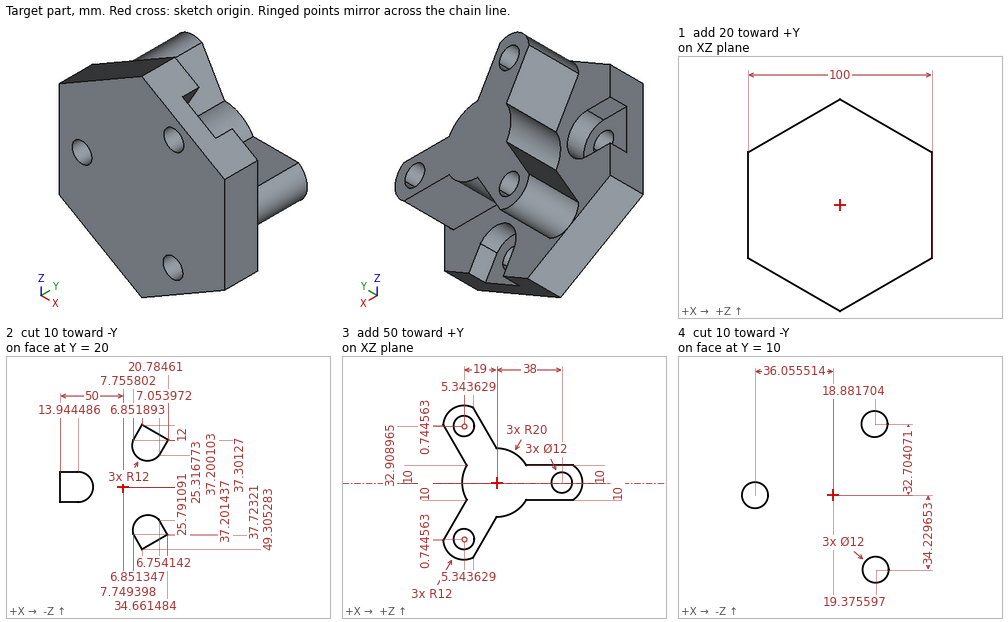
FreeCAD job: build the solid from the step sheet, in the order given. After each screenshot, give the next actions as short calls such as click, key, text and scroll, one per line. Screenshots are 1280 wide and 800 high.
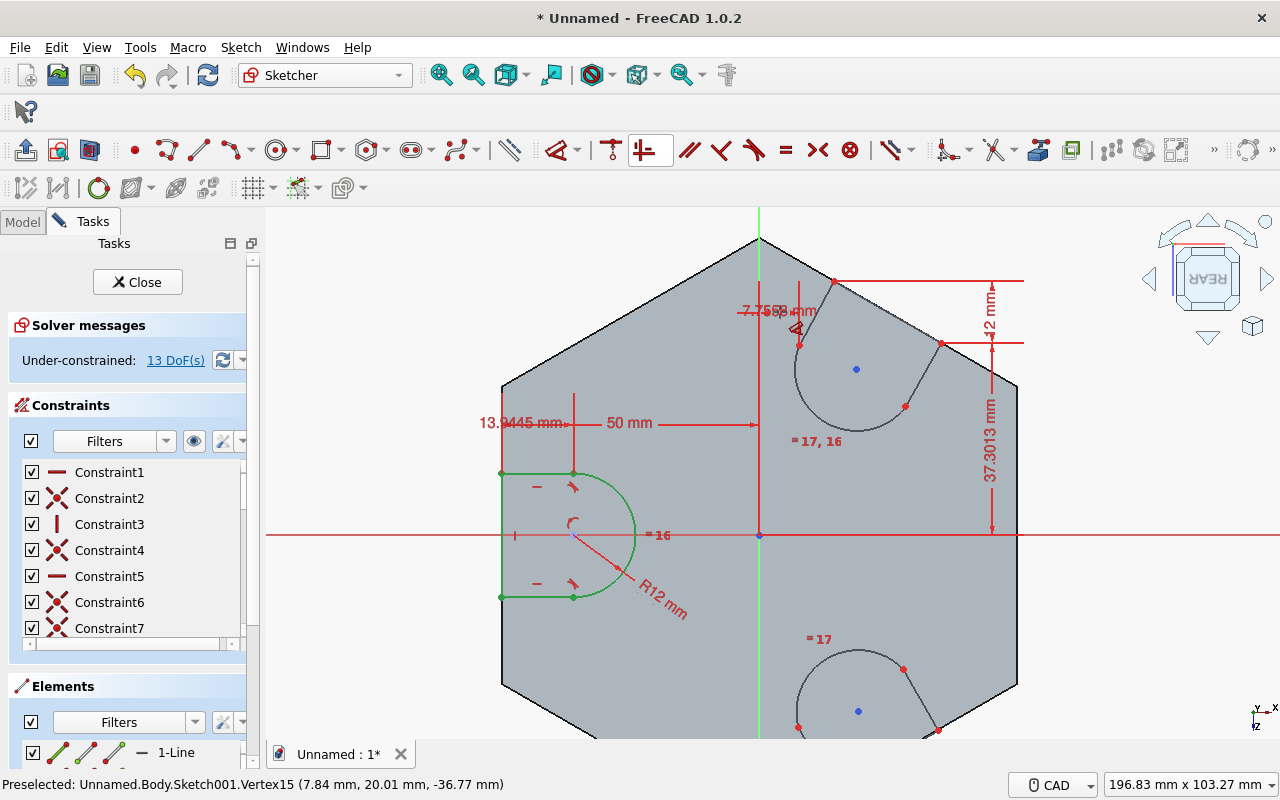
scroll(669, 346, down, 2)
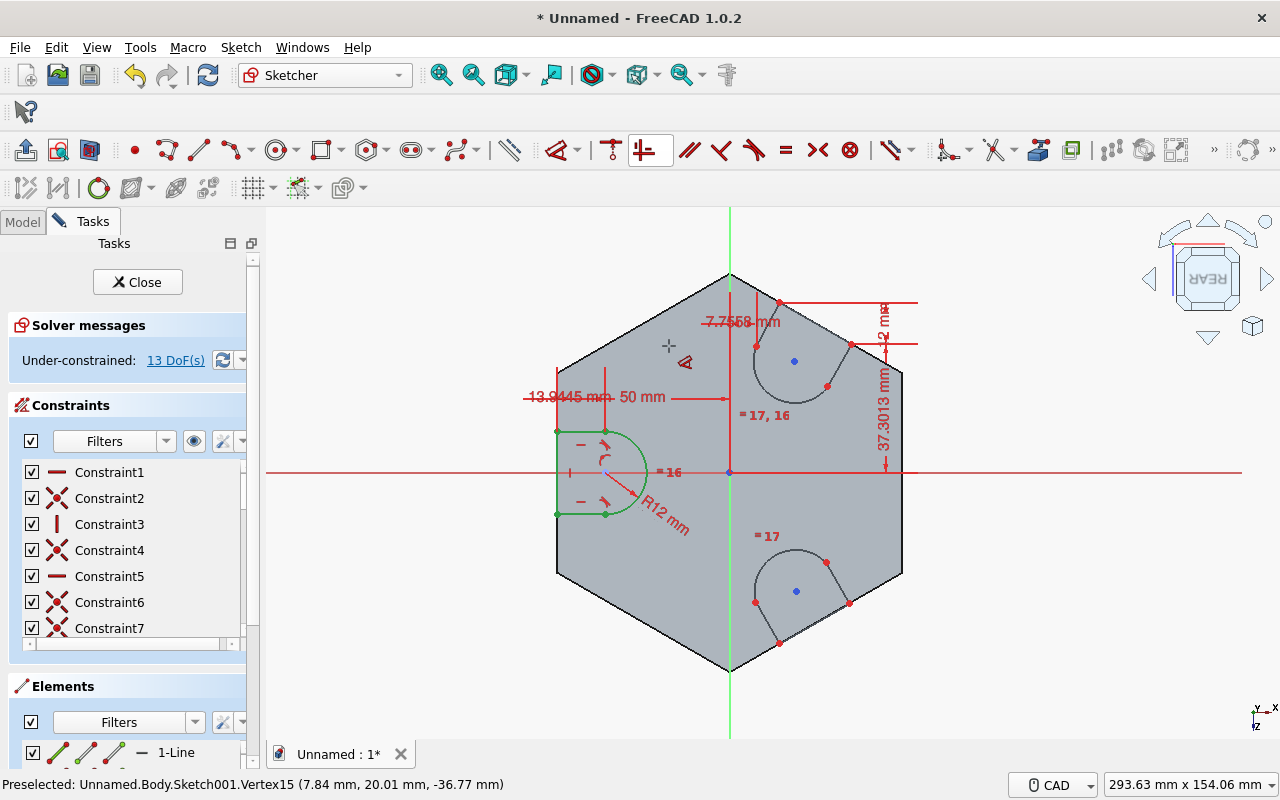
scroll(756, 602, up, 2)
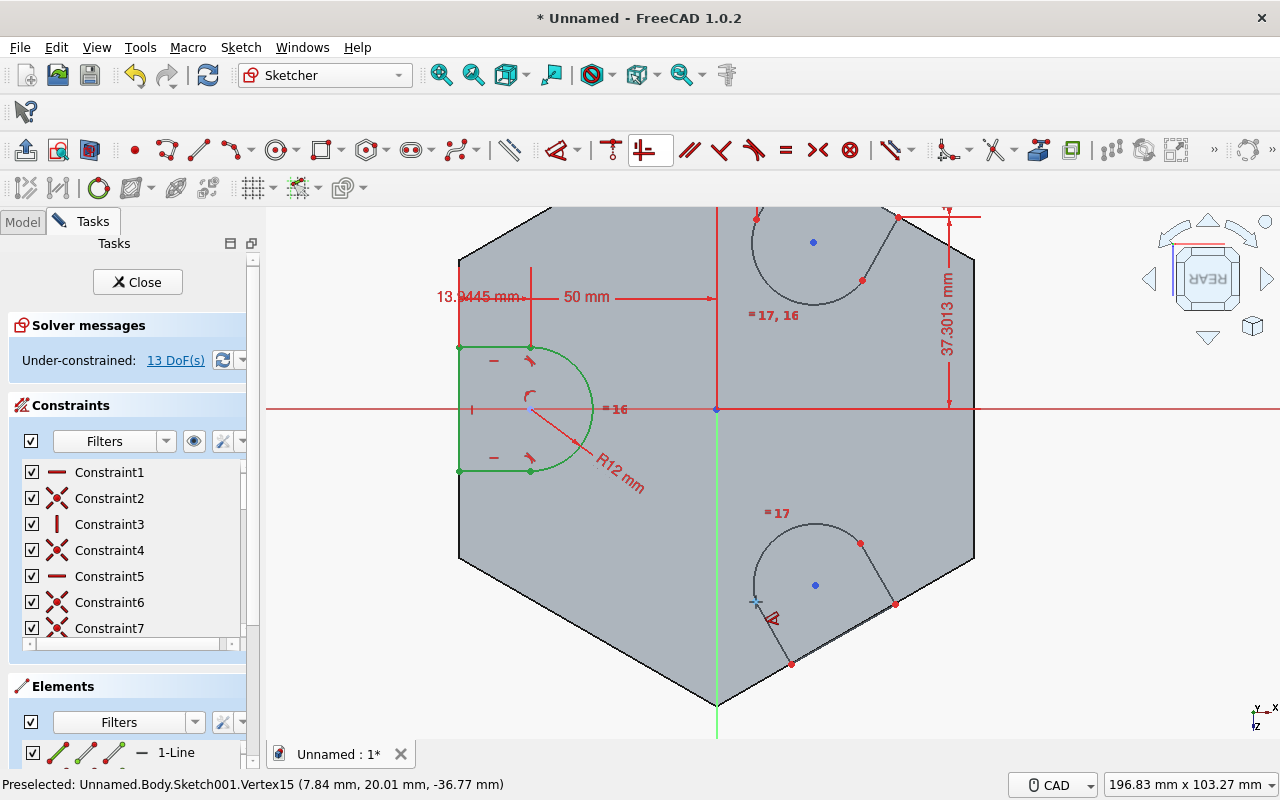
click(756, 602)
click(736, 636)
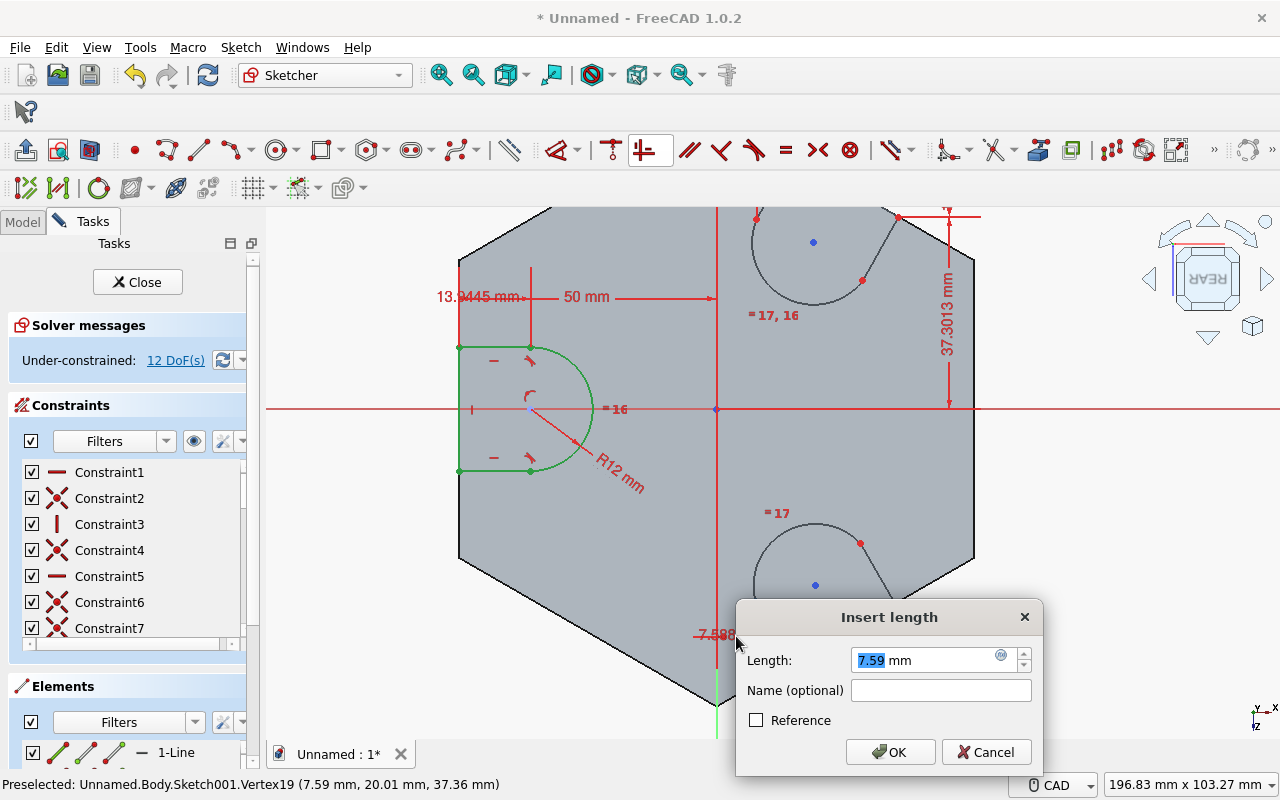
text(7.749398)
key(Return)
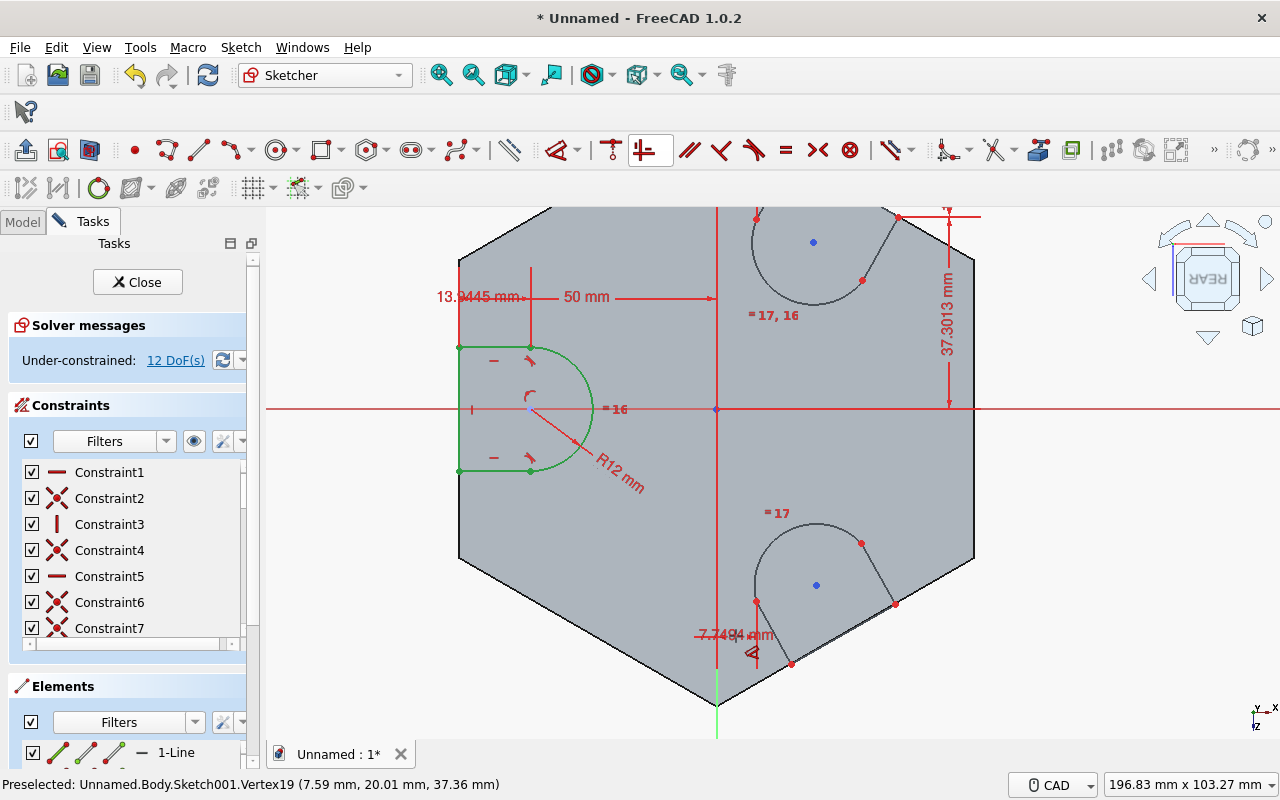
click(896, 605)
click(930, 507)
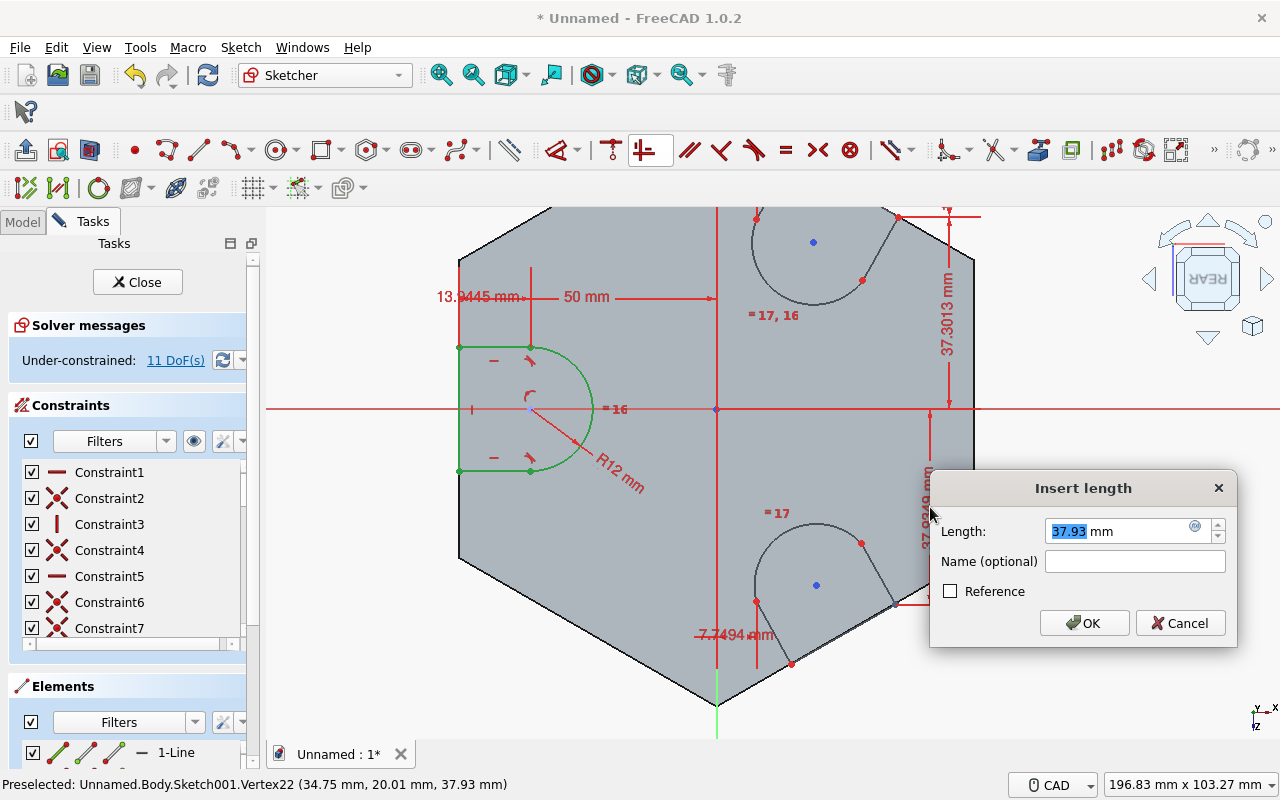
text(37.72321)
key(Return)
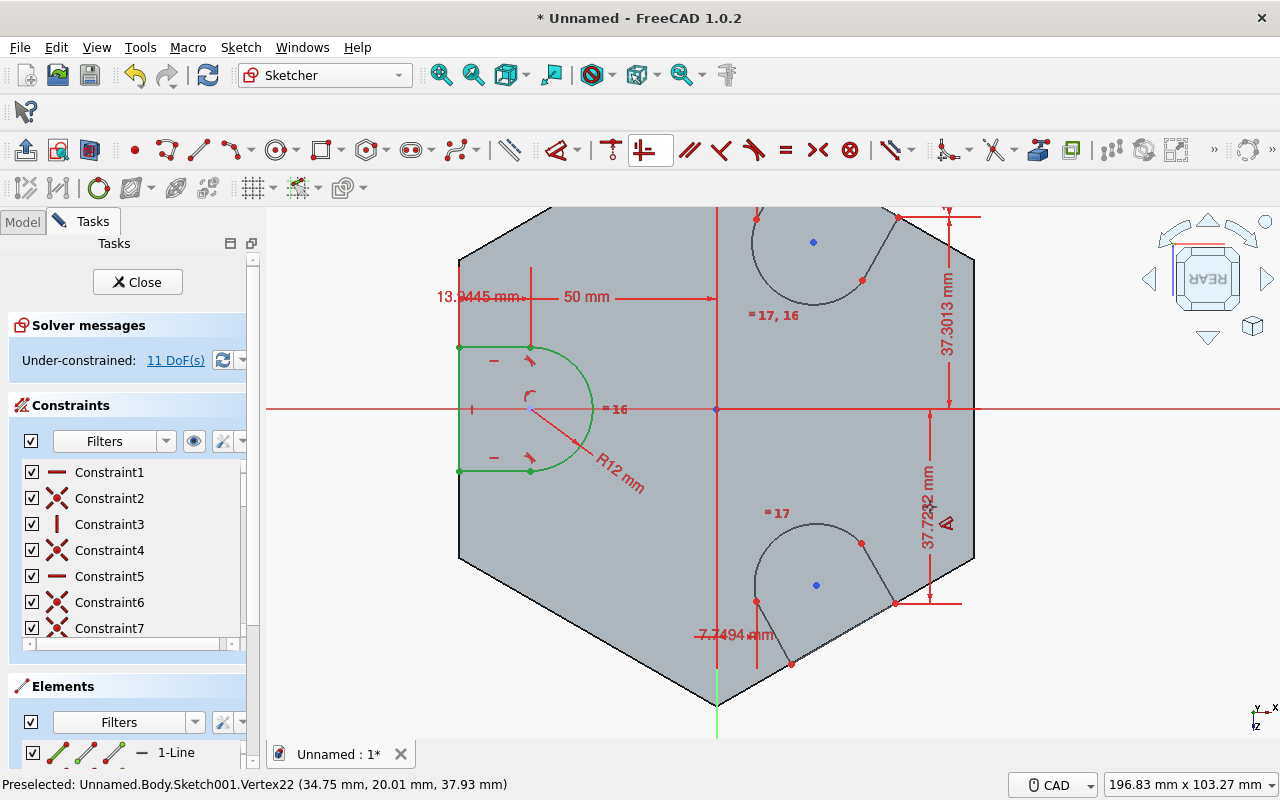
click(874, 262)
click(872, 315)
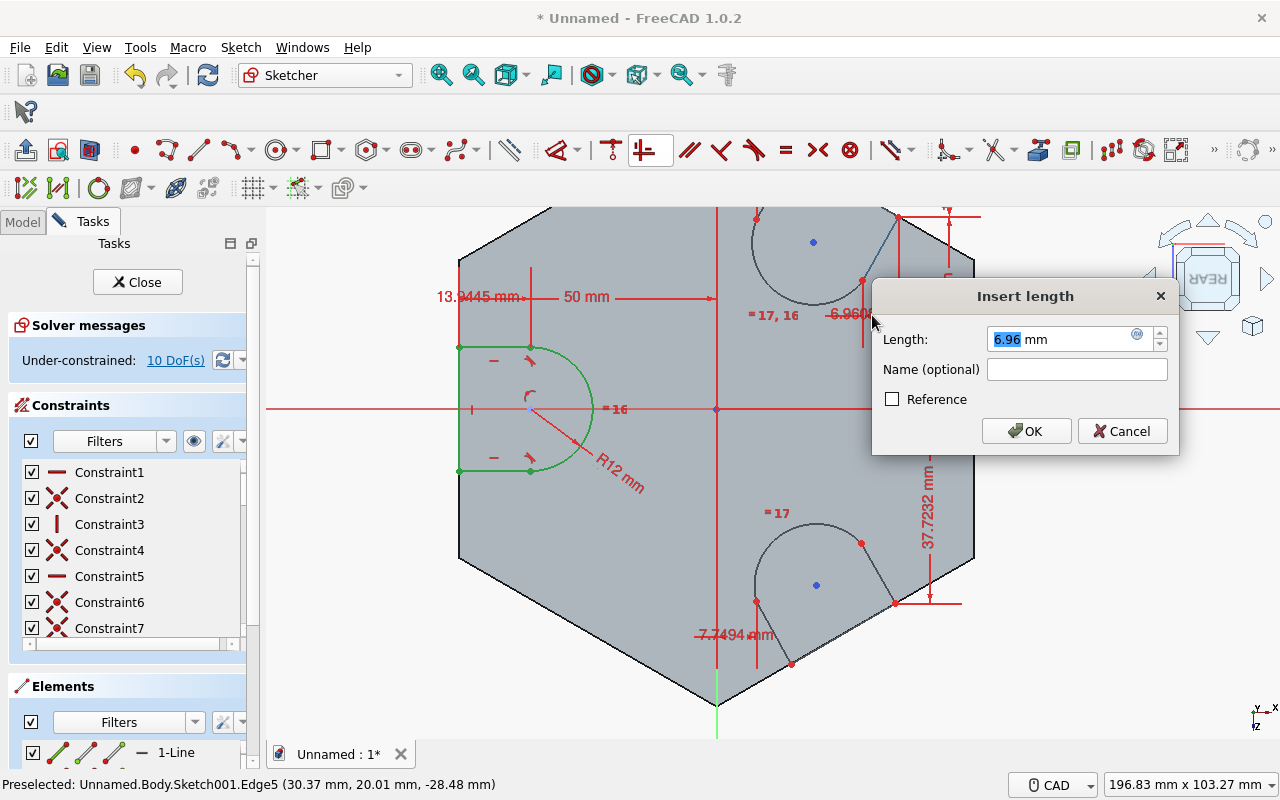
text(7.053972)
key(Return)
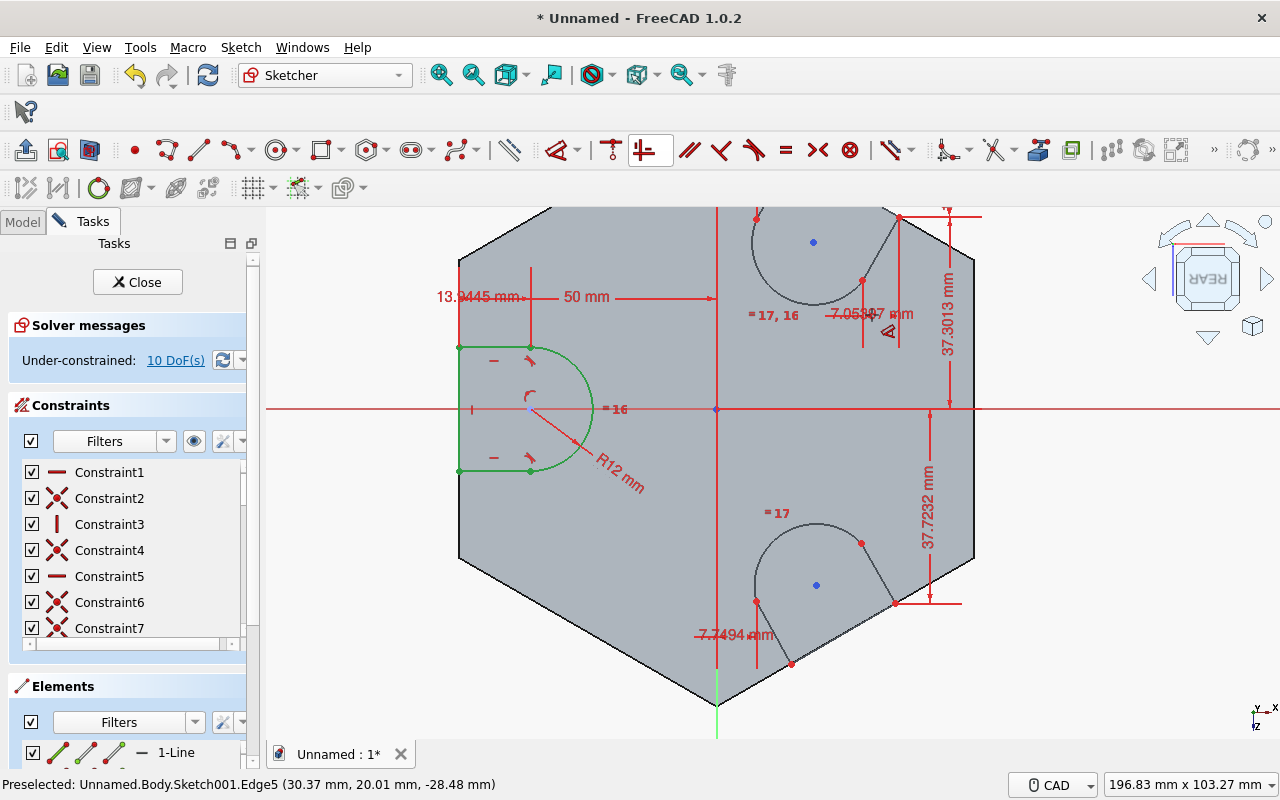
scroll(756, 603, down, 2)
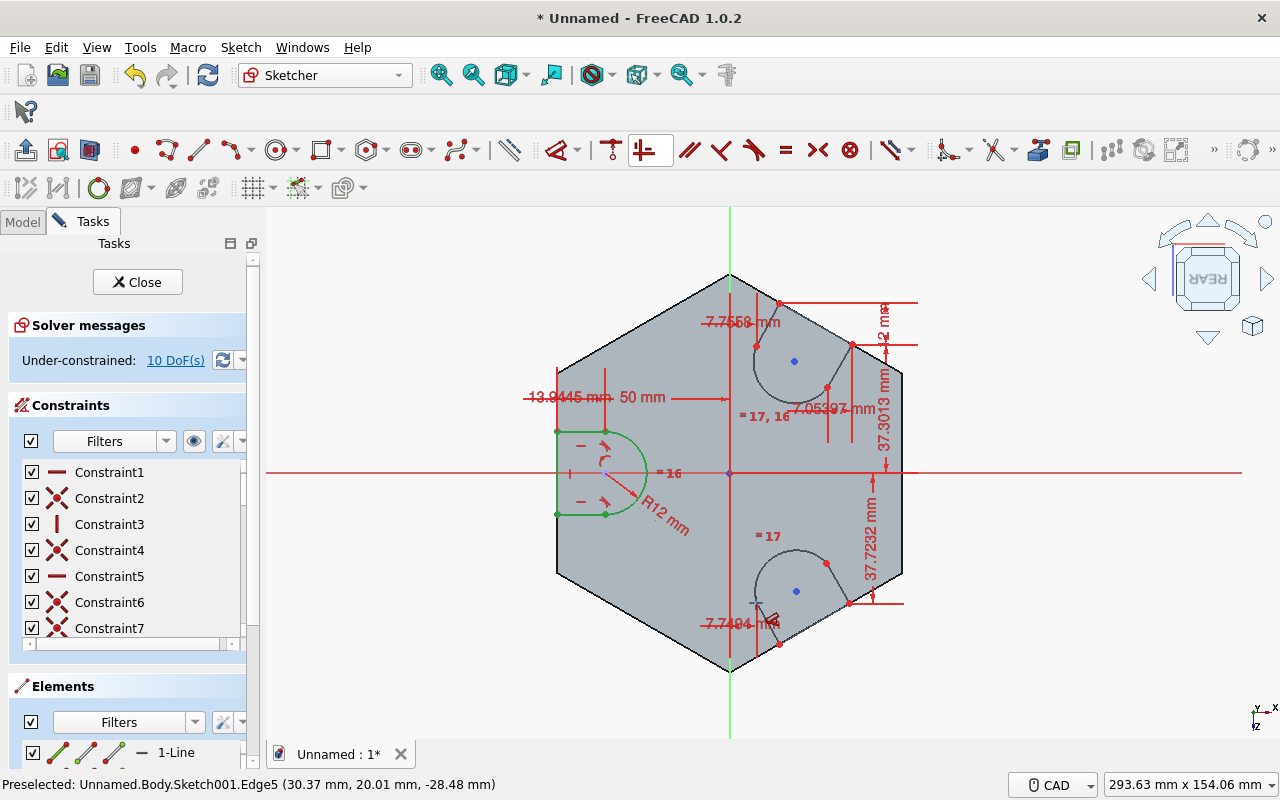
click(830, 332)
click(816, 269)